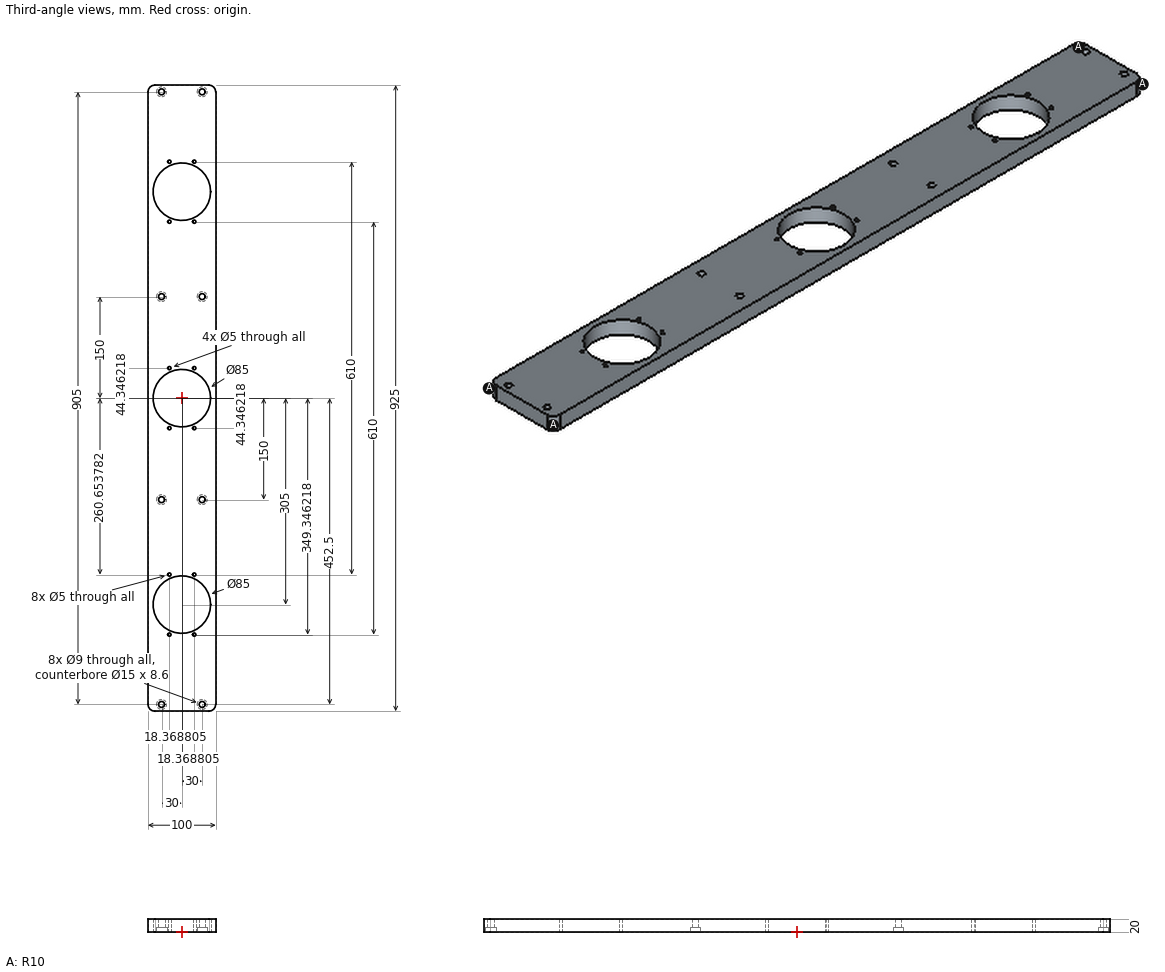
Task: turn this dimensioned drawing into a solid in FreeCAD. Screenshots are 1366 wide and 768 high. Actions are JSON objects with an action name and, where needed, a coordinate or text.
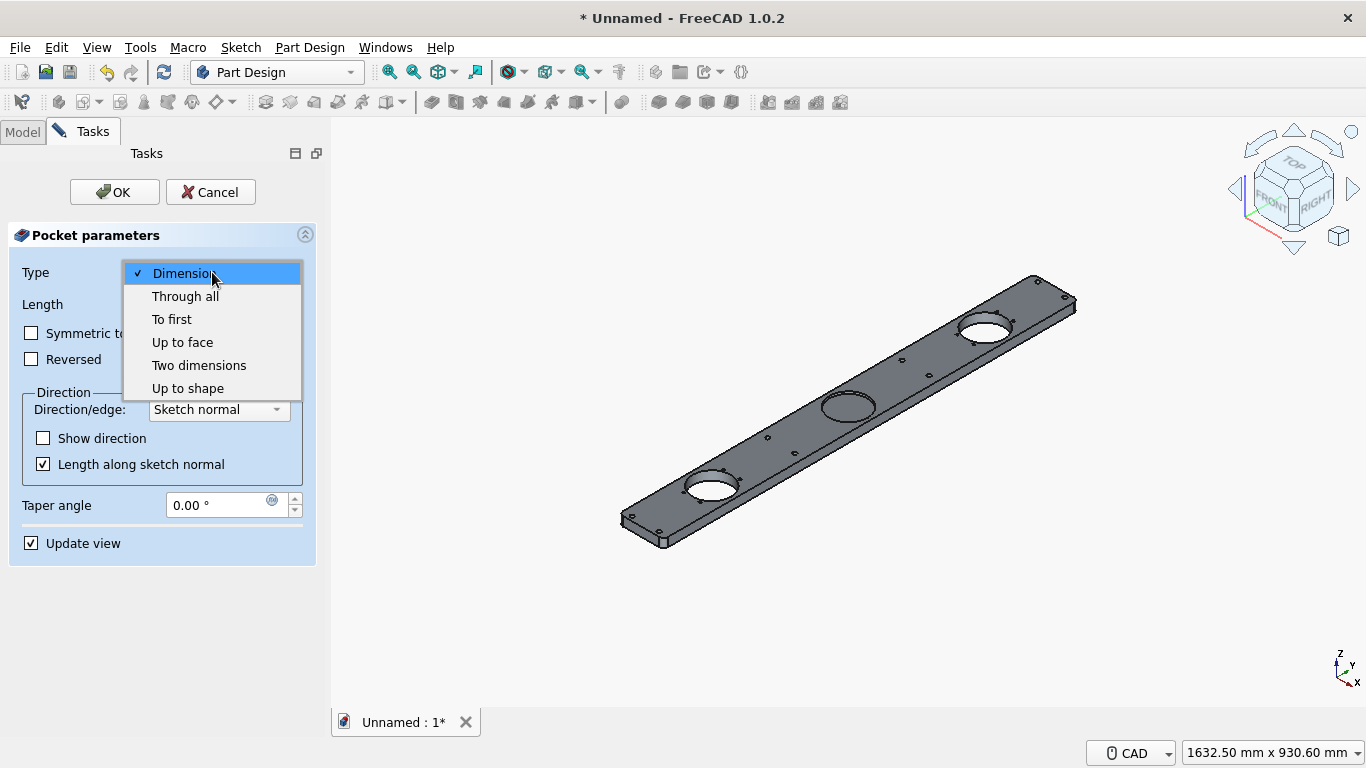
{"action": "left_click", "coordinate": [212, 296]}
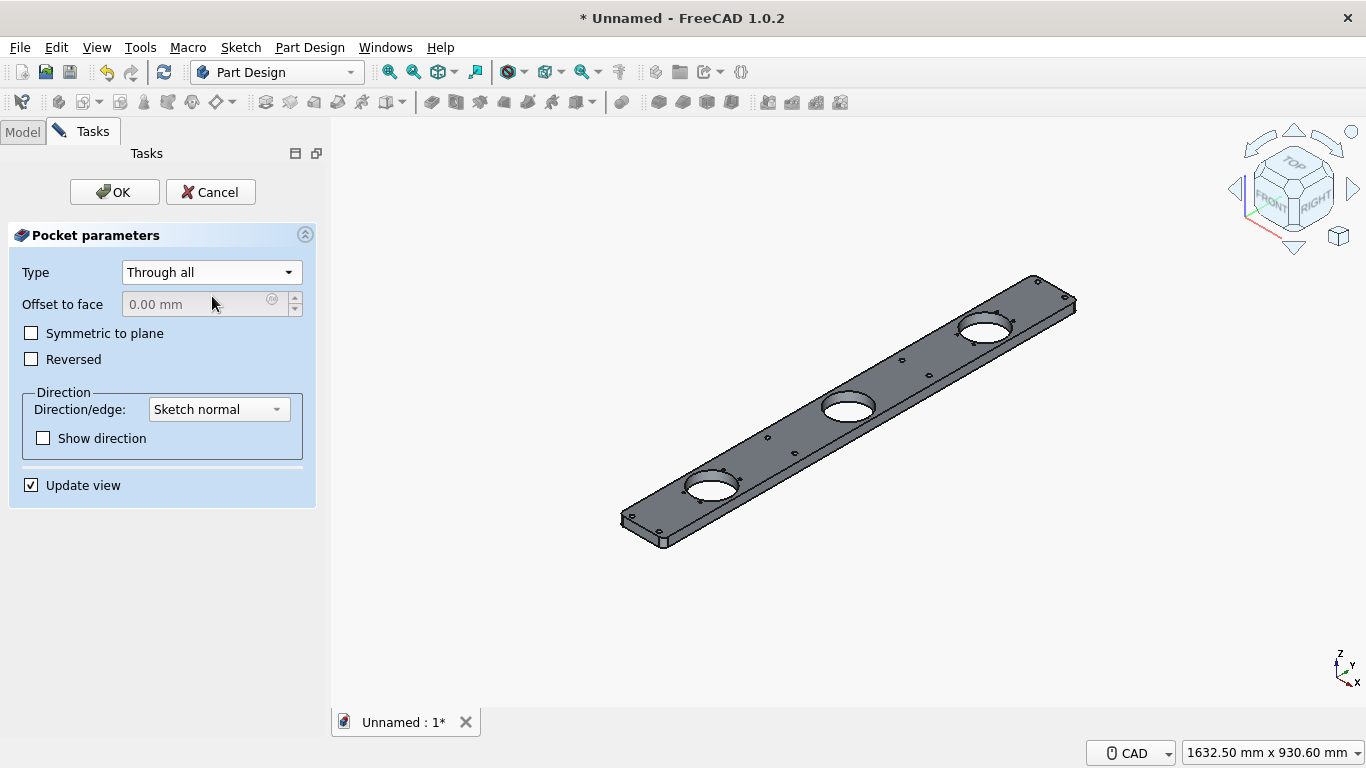
{"action": "left_click", "coordinate": [115, 192]}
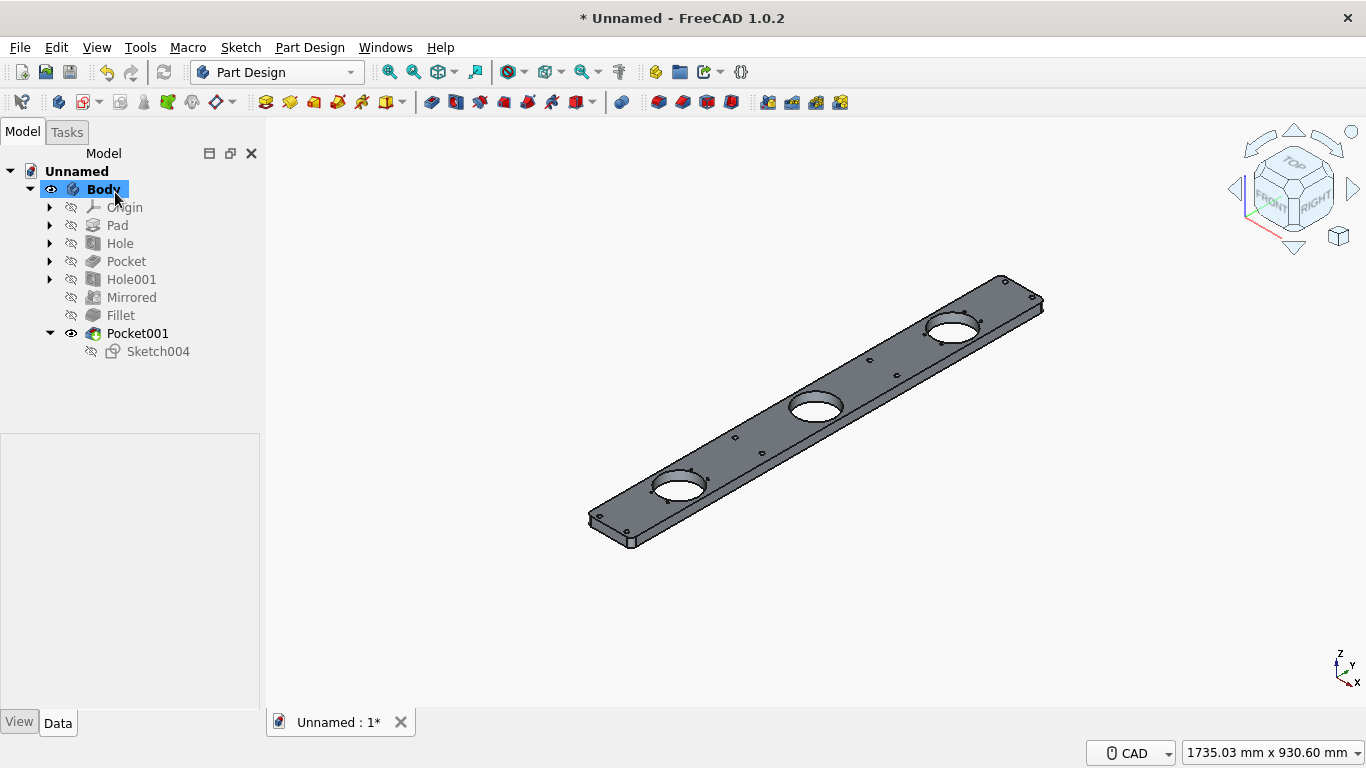
{"action": "left_click", "coordinate": [638, 508]}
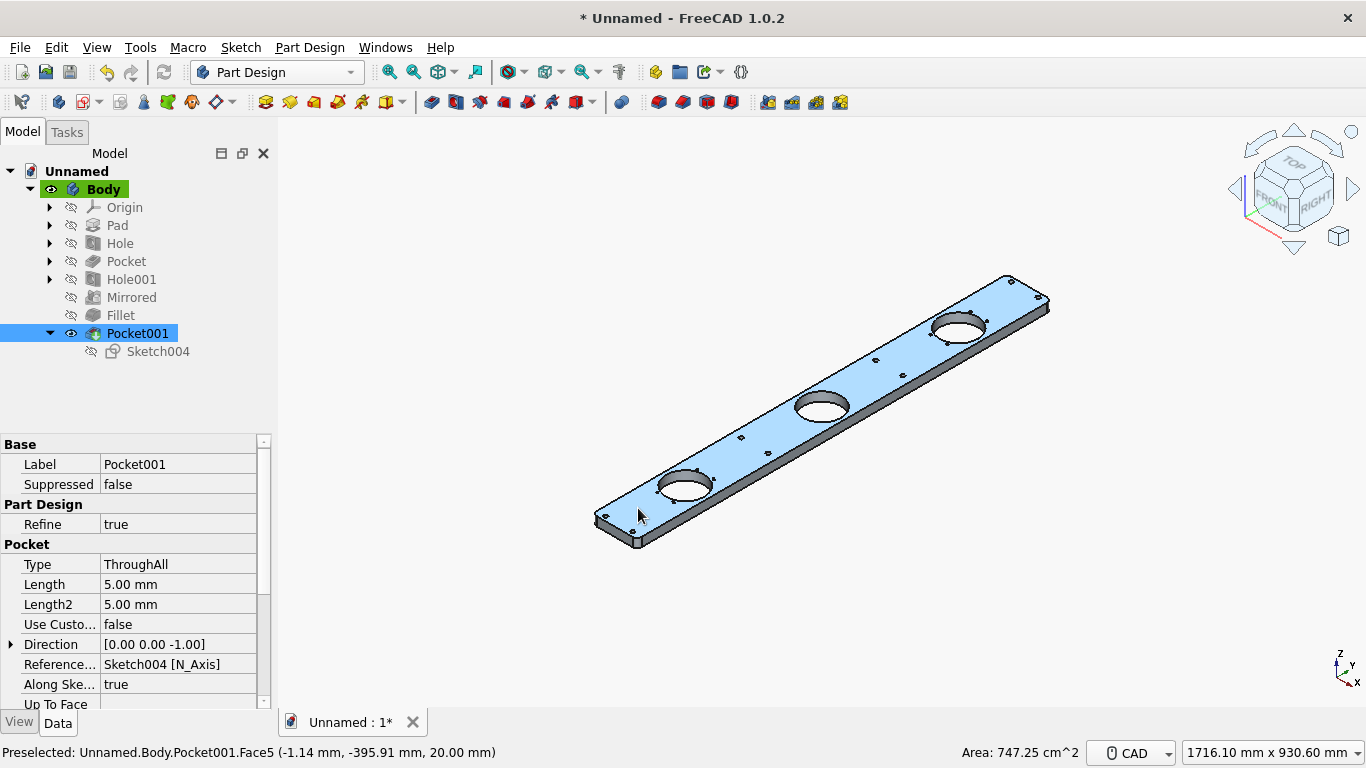
{"action": "left_click", "coordinate": [84, 102]}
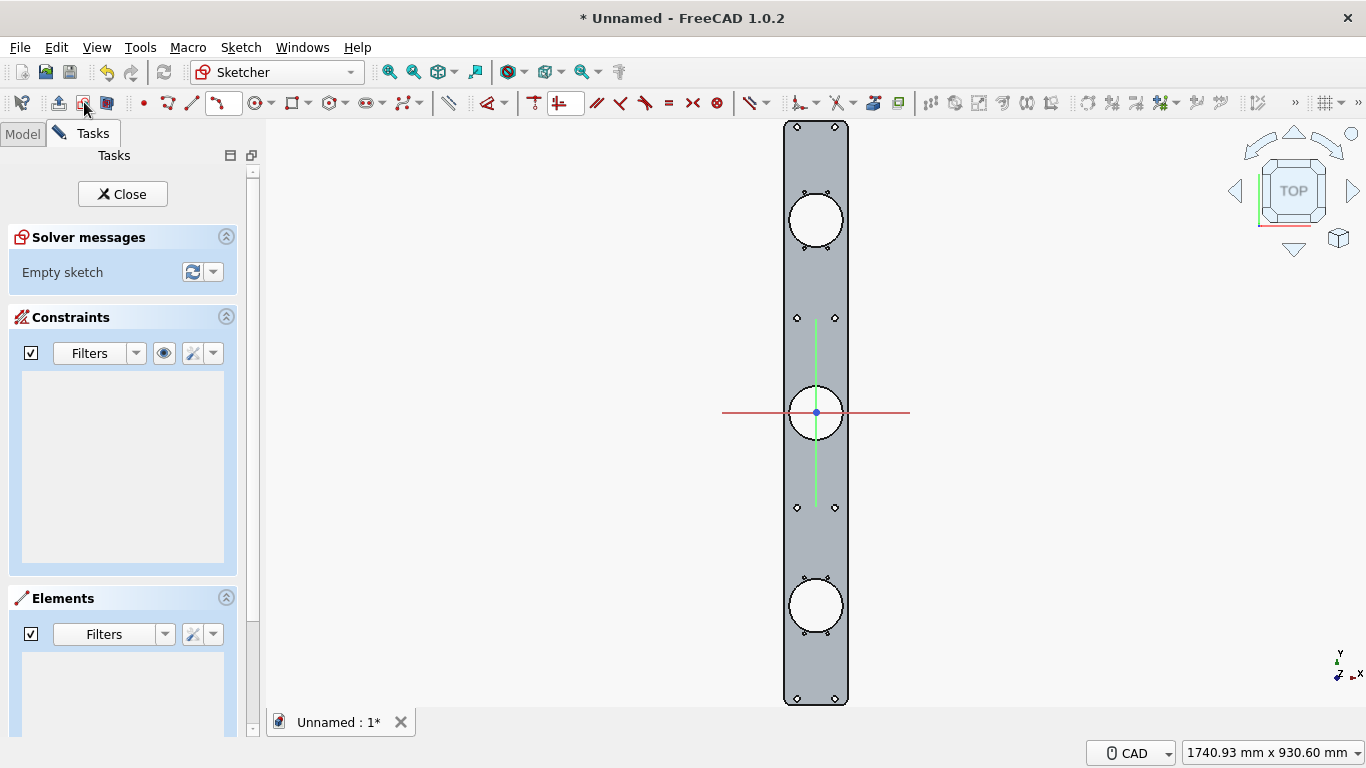
{"action": "scroll", "coordinate": [830, 413], "scroll_direction": "up", "scroll_amount": 9}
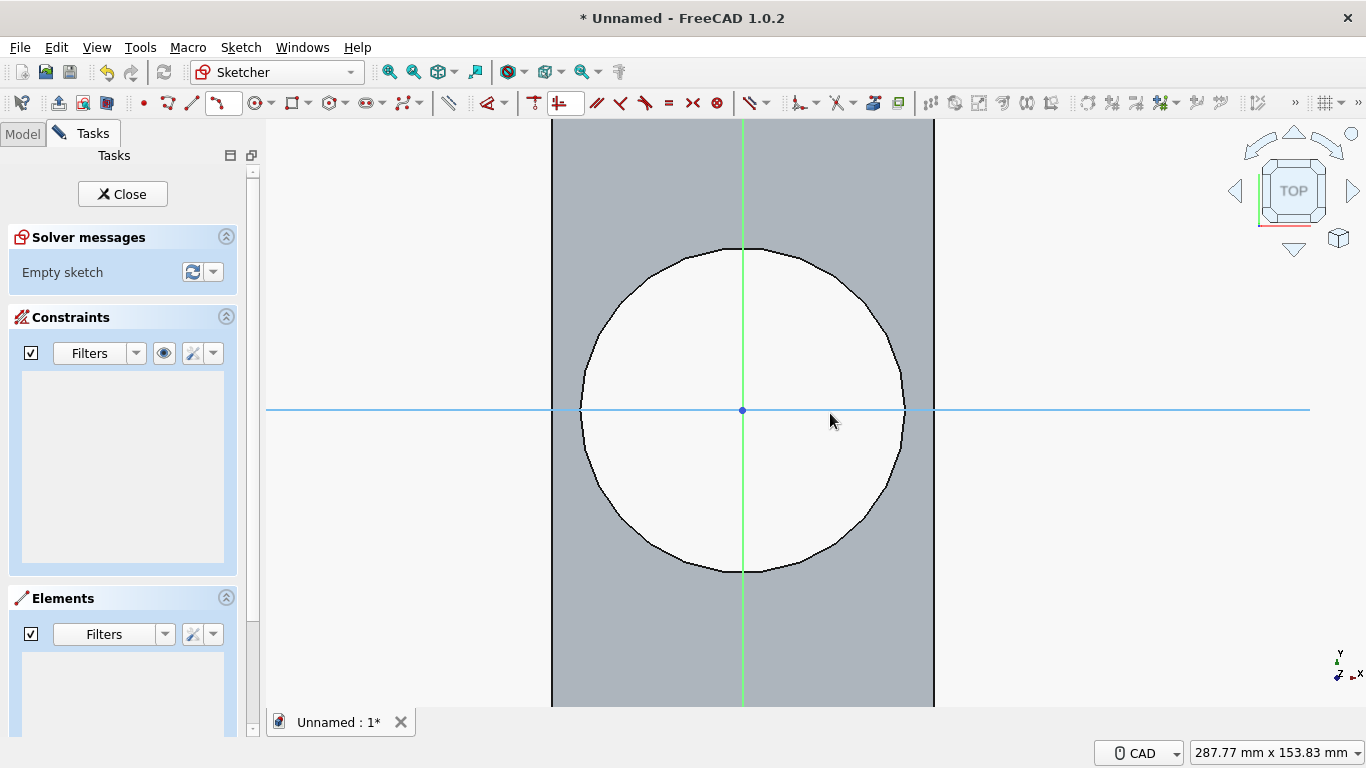
{"action": "key", "text": "g c"}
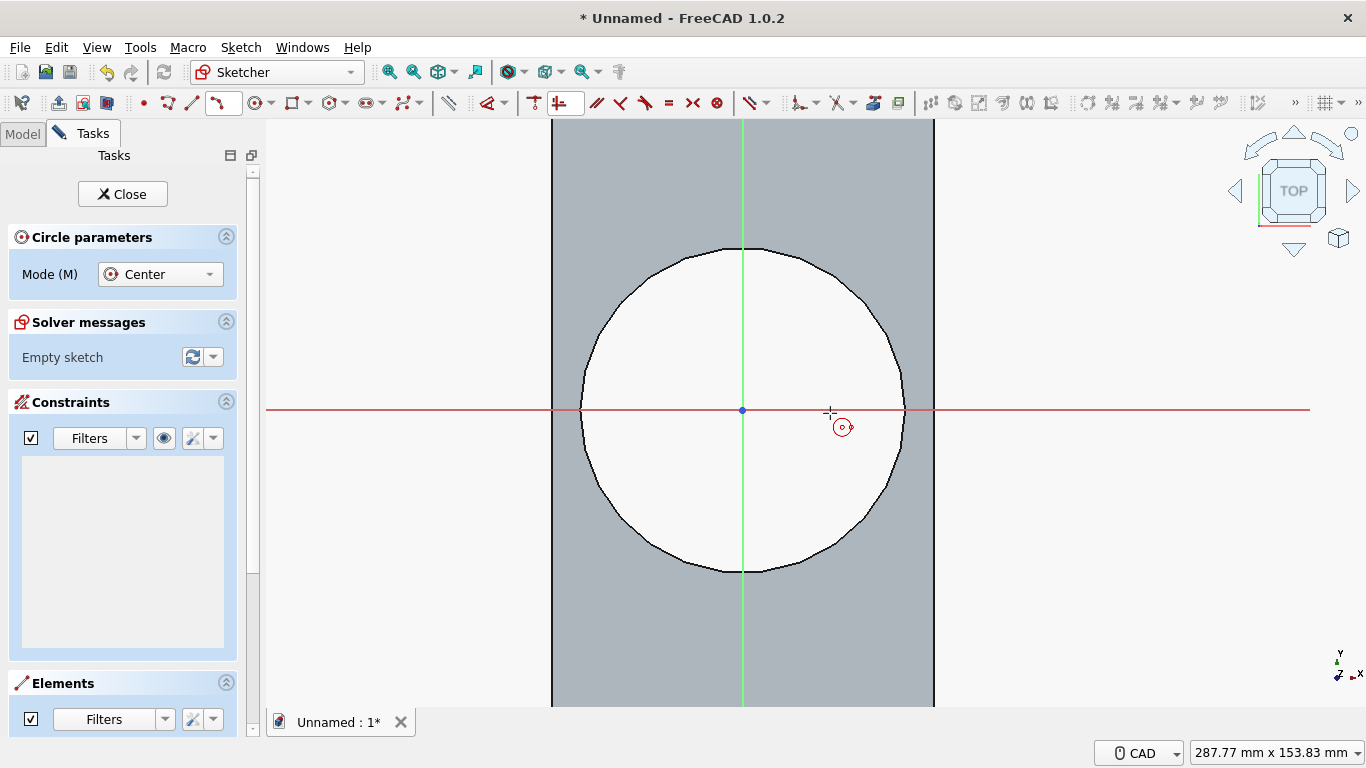
{"action": "scroll", "coordinate": [672, 241], "scroll_direction": "up", "scroll_amount": 5}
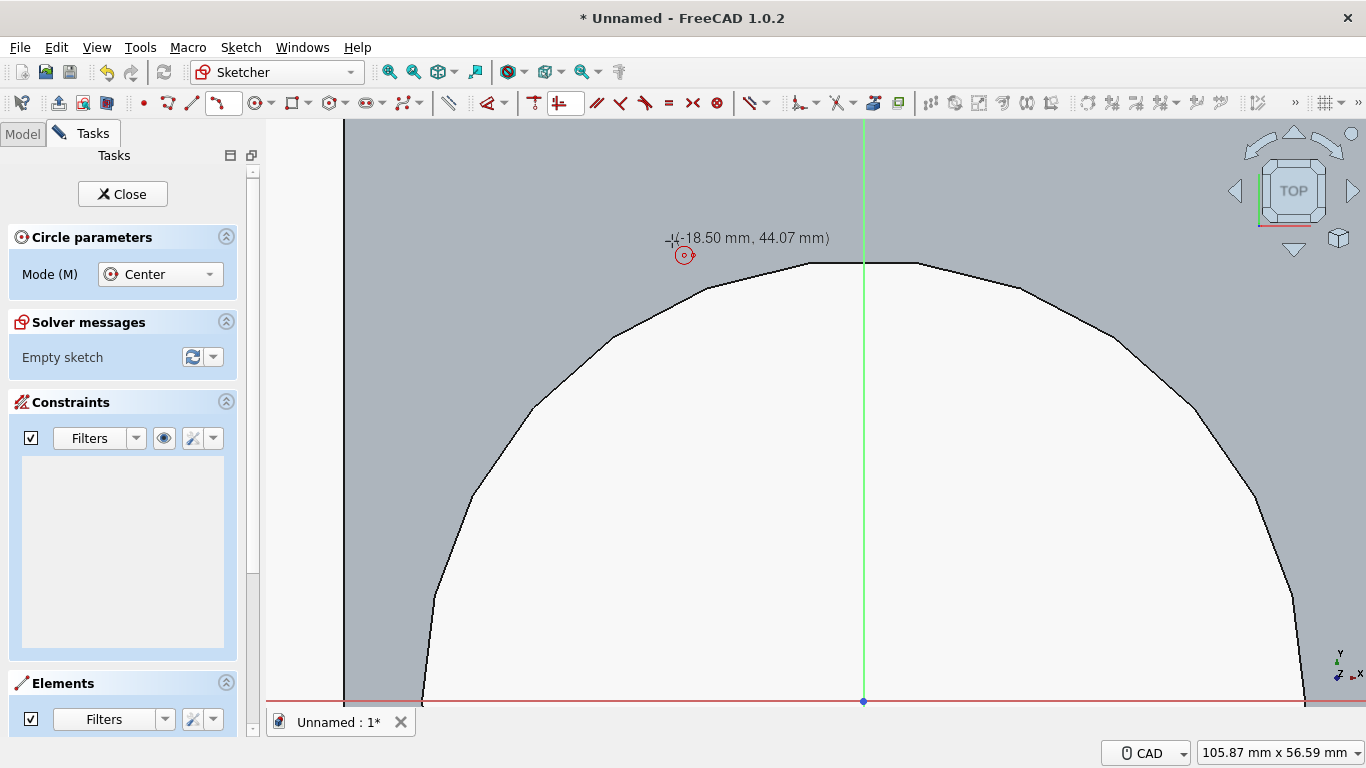
{"action": "left_click", "coordinate": [673, 241]}
{"action": "left_click", "coordinate": [691, 222]}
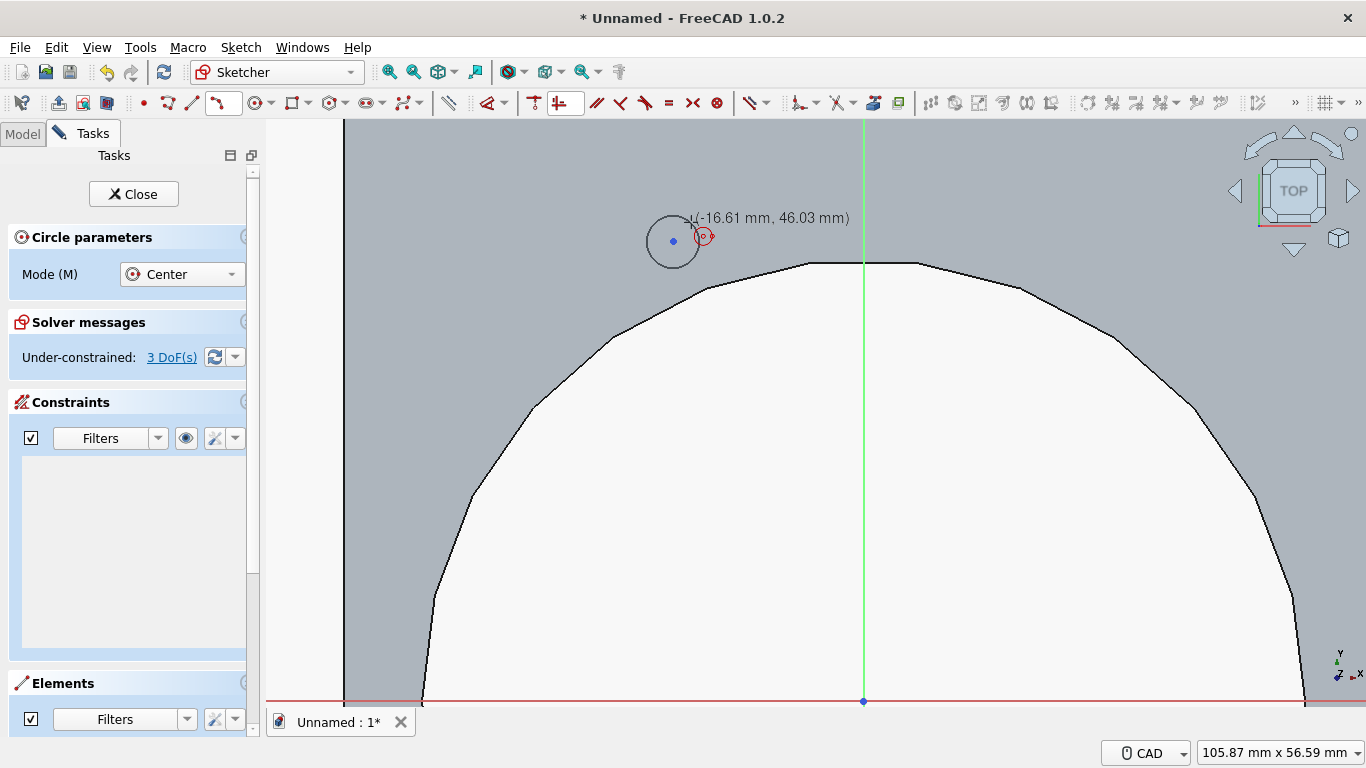
{"action": "left_click", "coordinate": [1054, 241]}
{"action": "left_click", "coordinate": [1073, 222]}